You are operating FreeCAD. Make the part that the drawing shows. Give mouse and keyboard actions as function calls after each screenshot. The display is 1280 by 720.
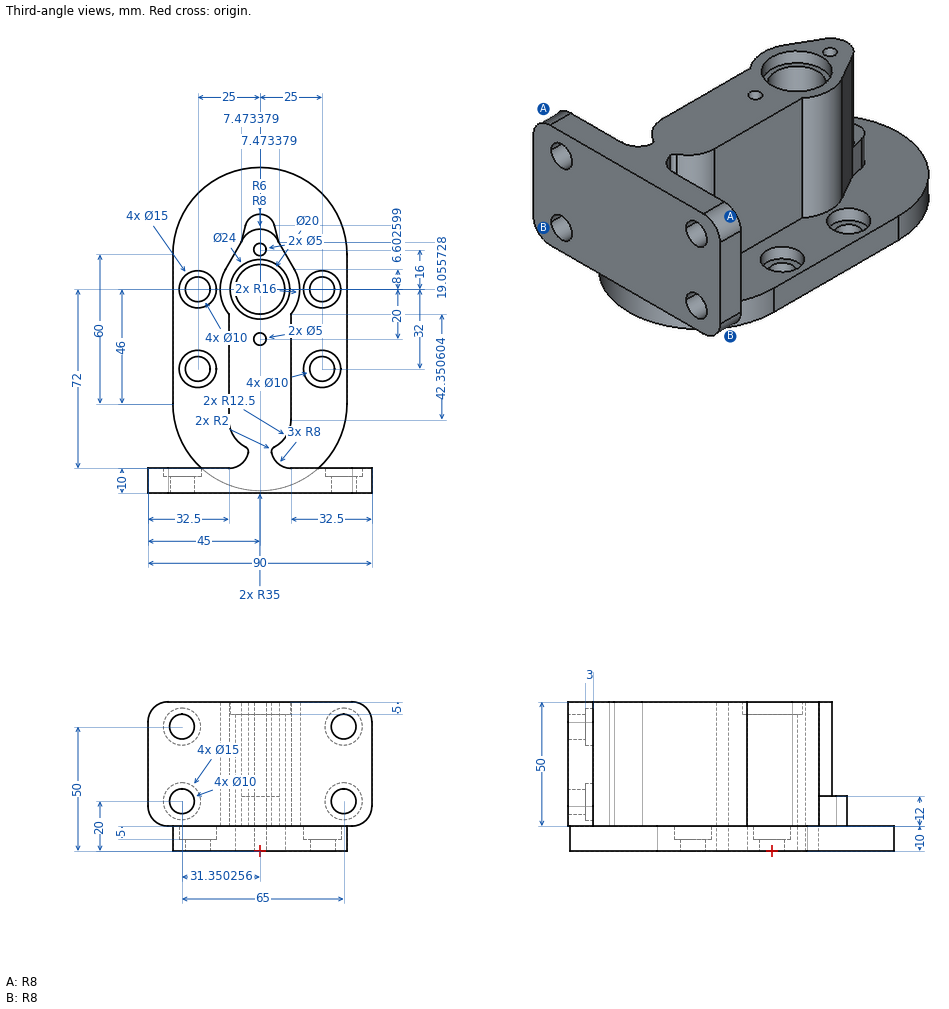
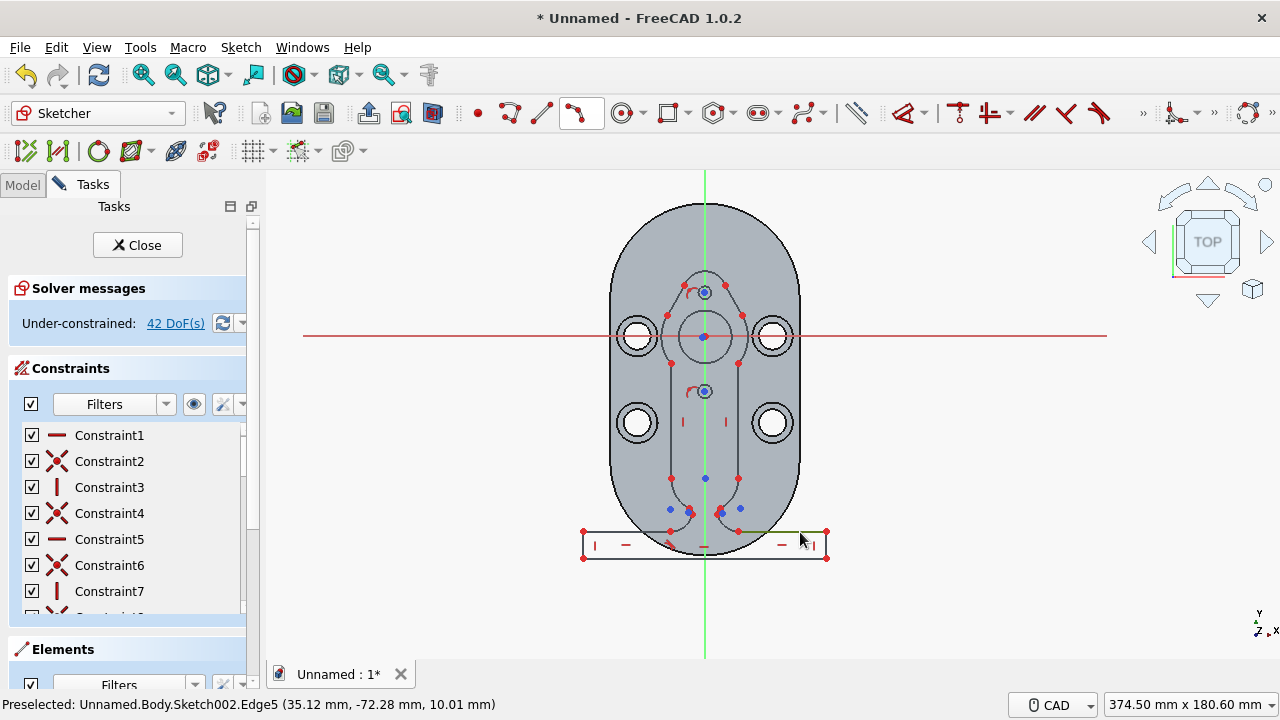
click(725, 527)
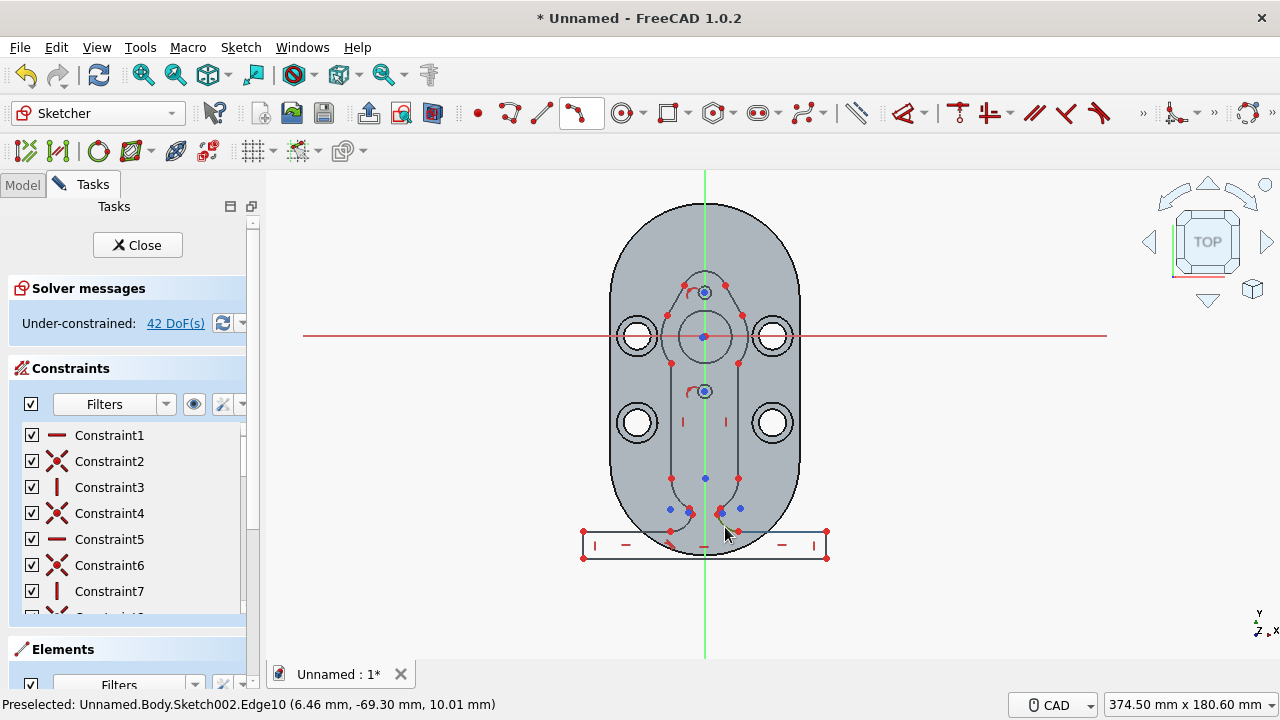
click(1100, 114)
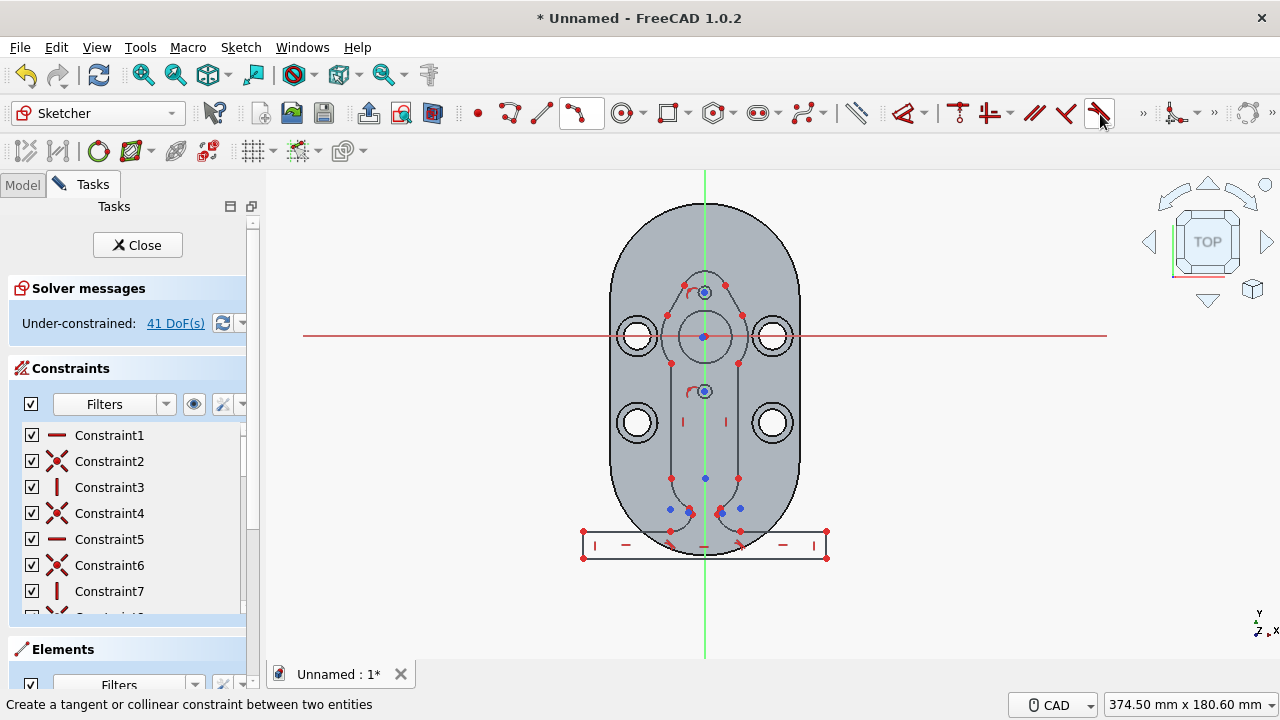
click(738, 444)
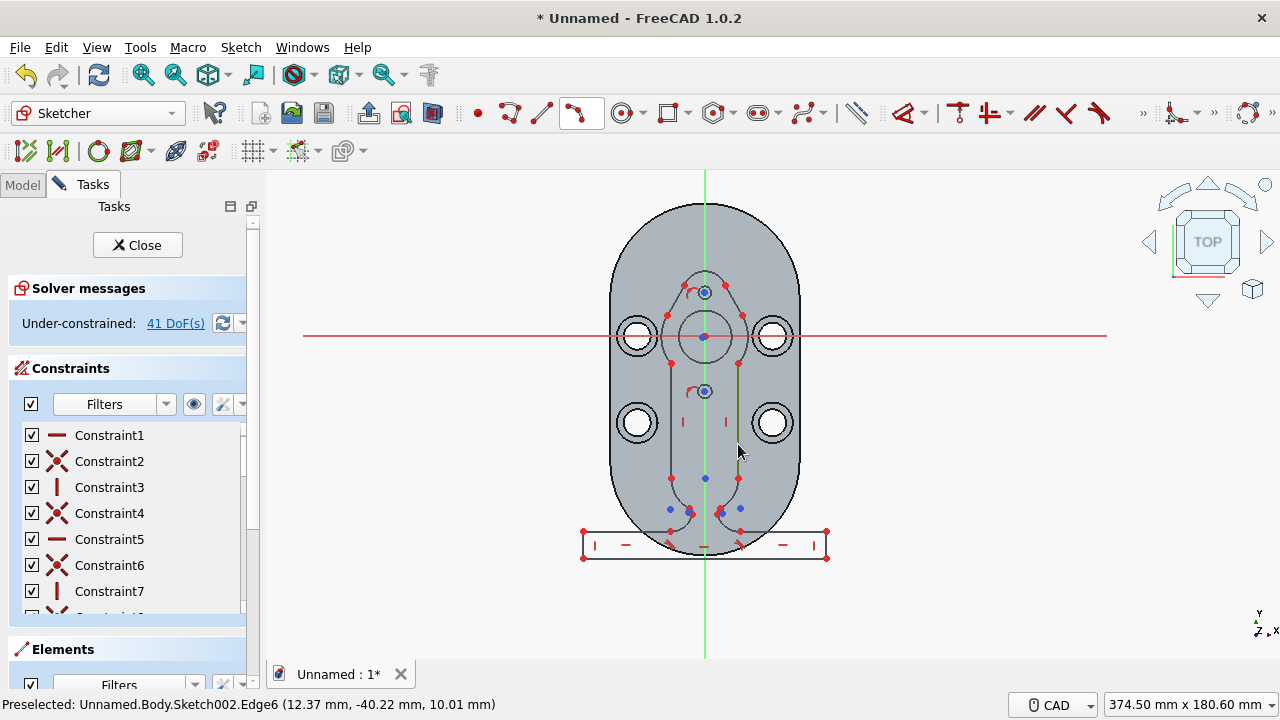
scroll(729, 502, up, 2)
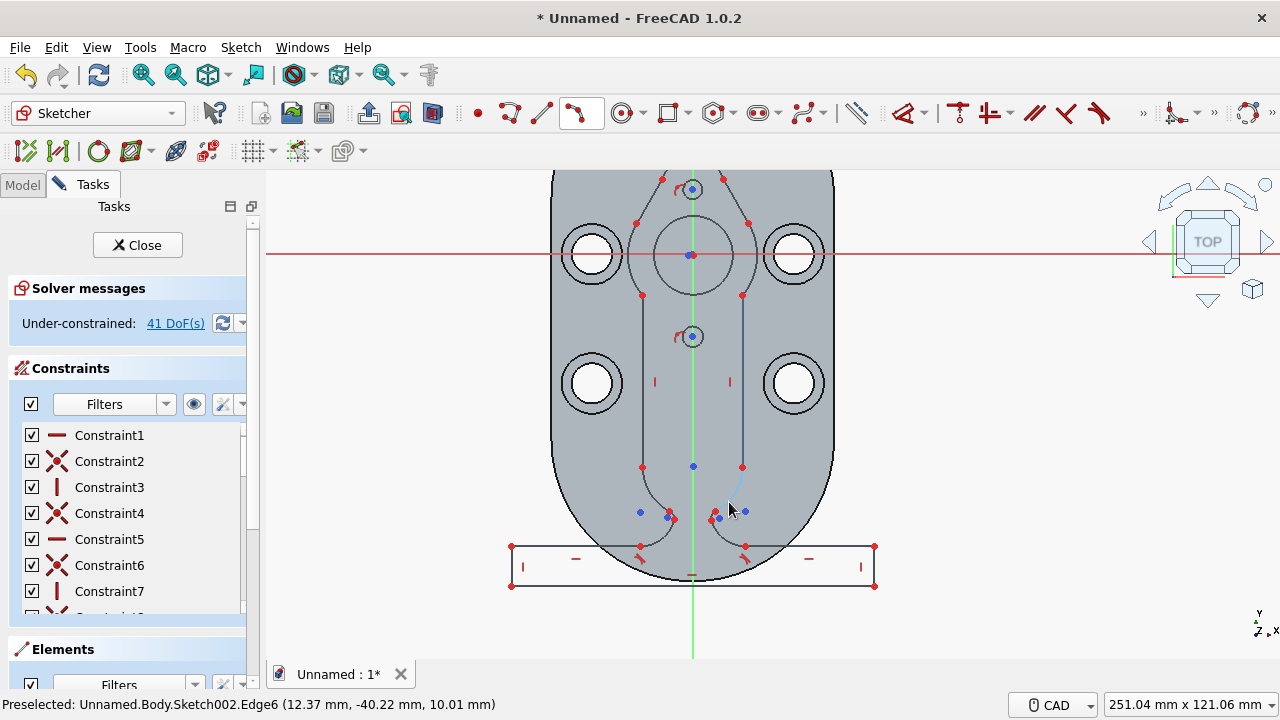
click(729, 501)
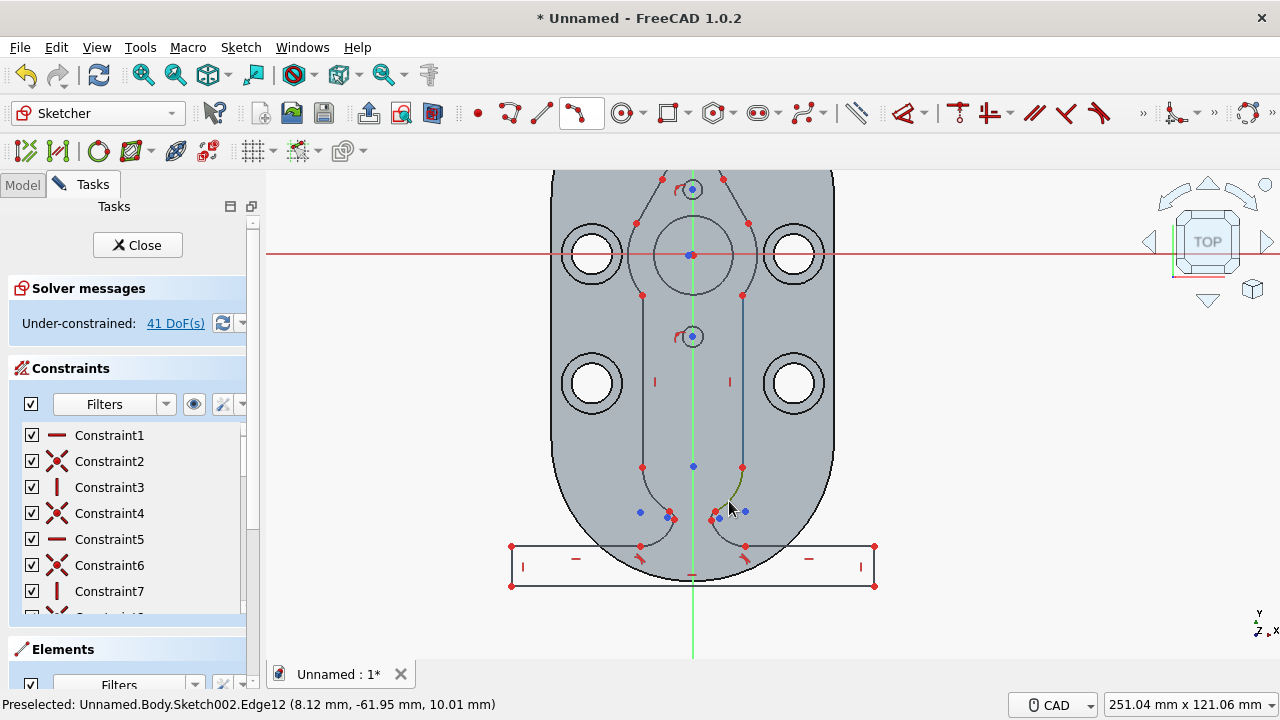
click(1100, 114)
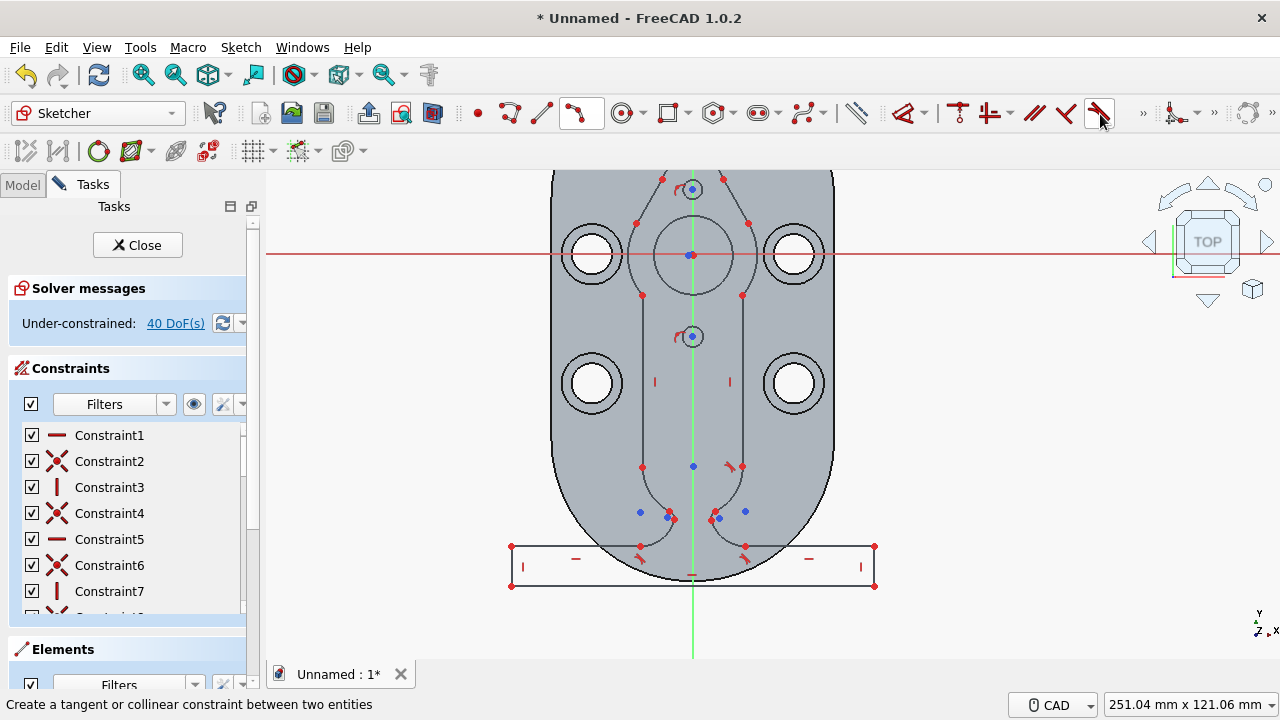
click(741, 210)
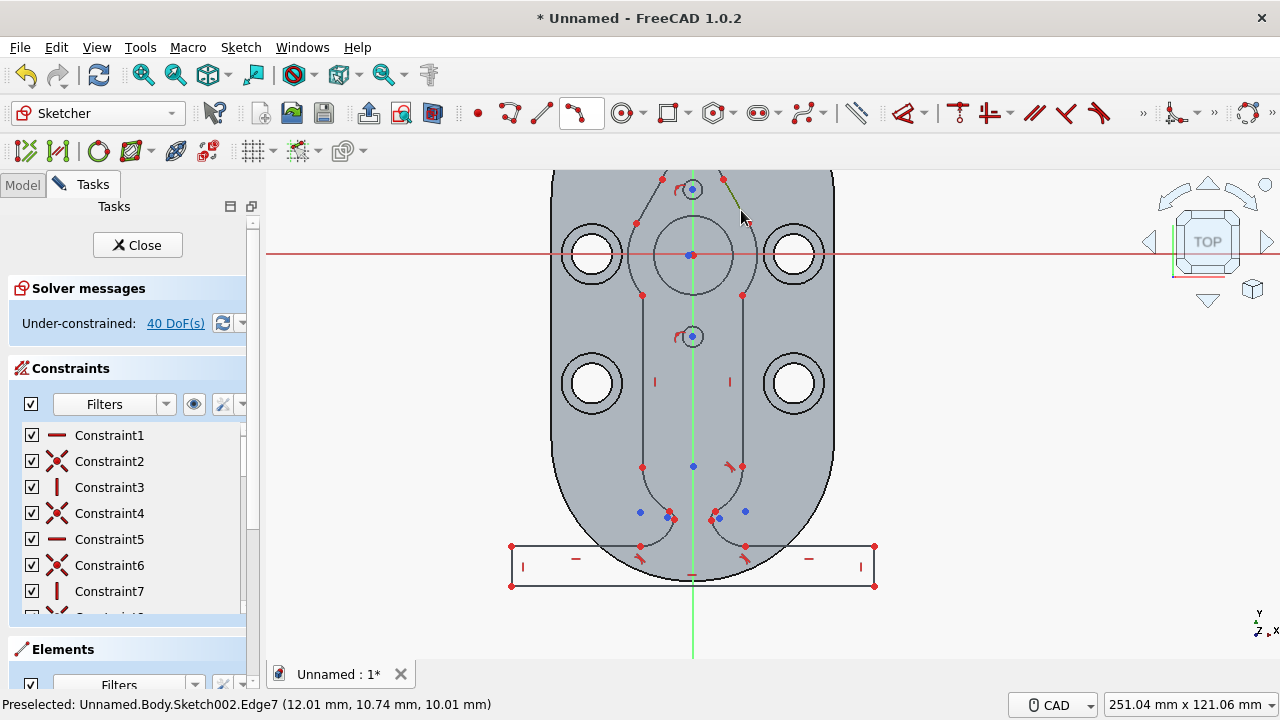
click(754, 276)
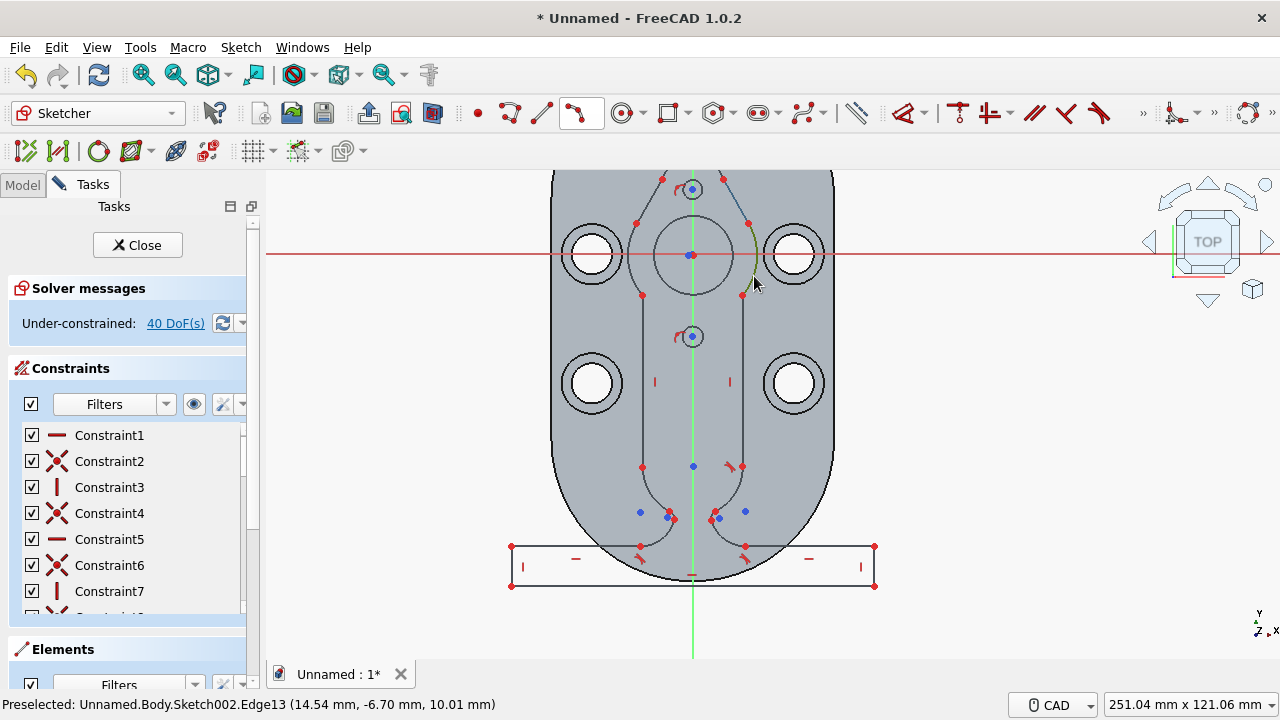
click(1100, 114)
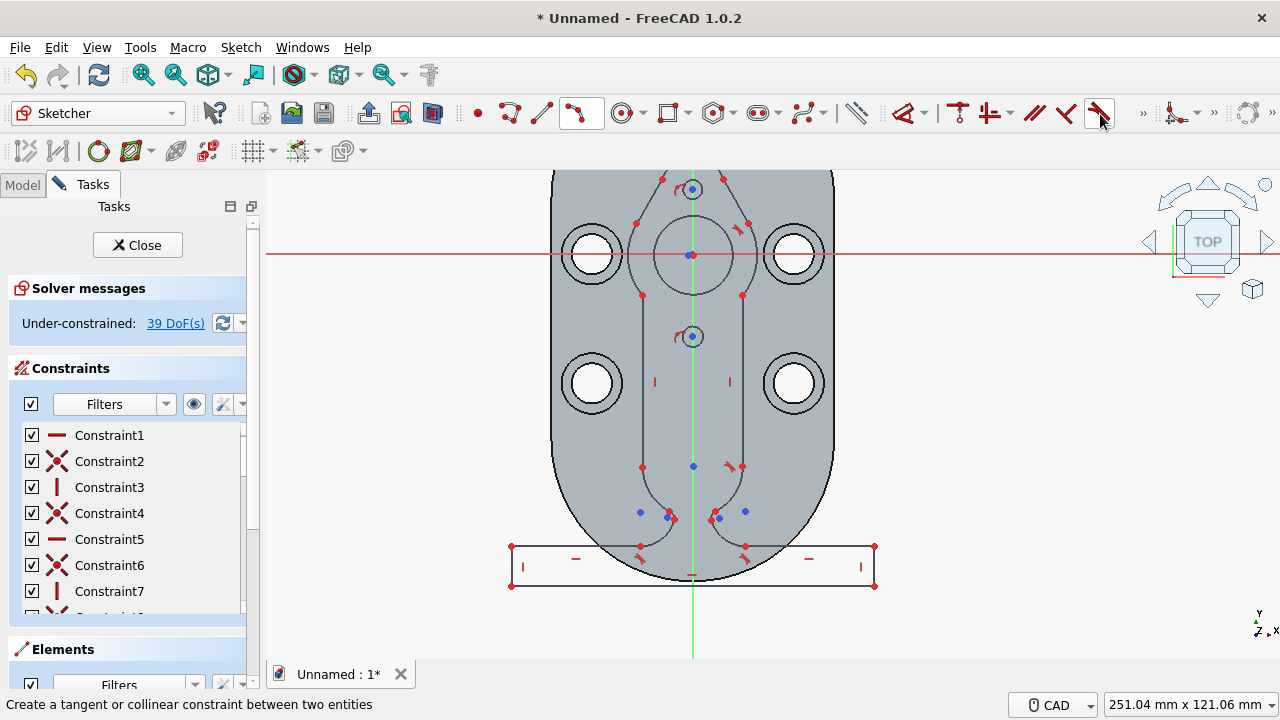
click(644, 210)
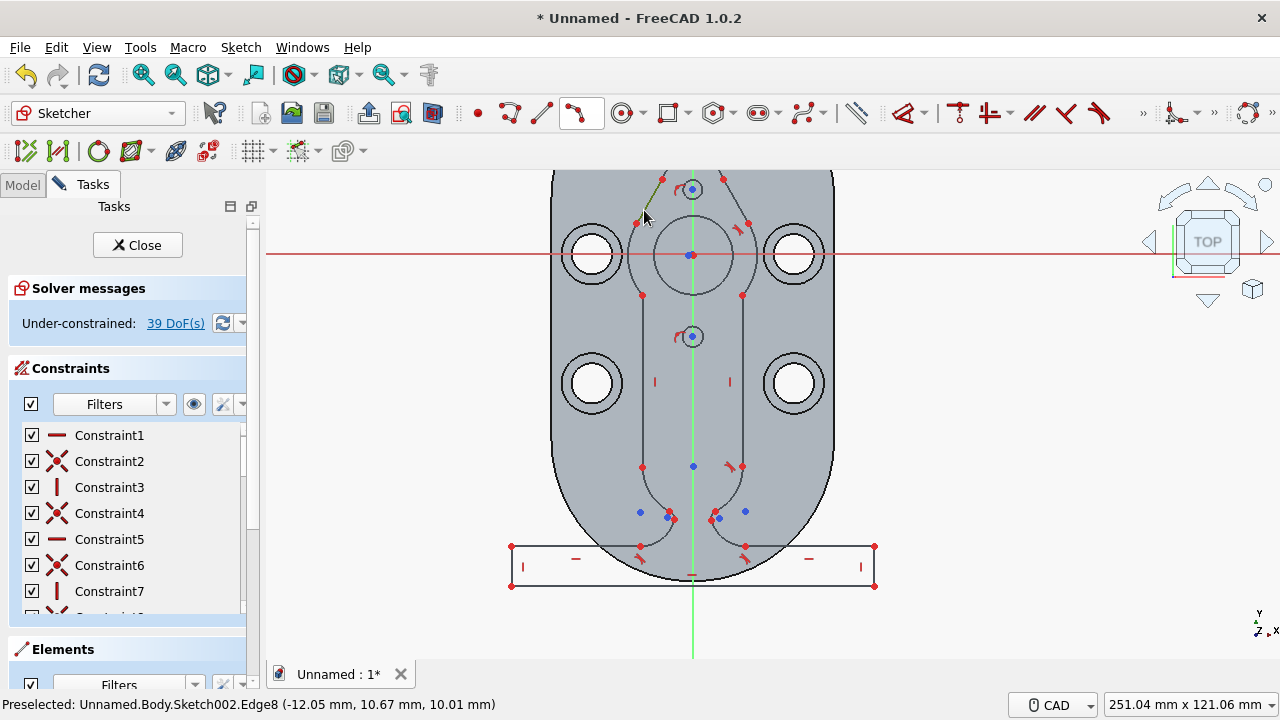
click(631, 276)